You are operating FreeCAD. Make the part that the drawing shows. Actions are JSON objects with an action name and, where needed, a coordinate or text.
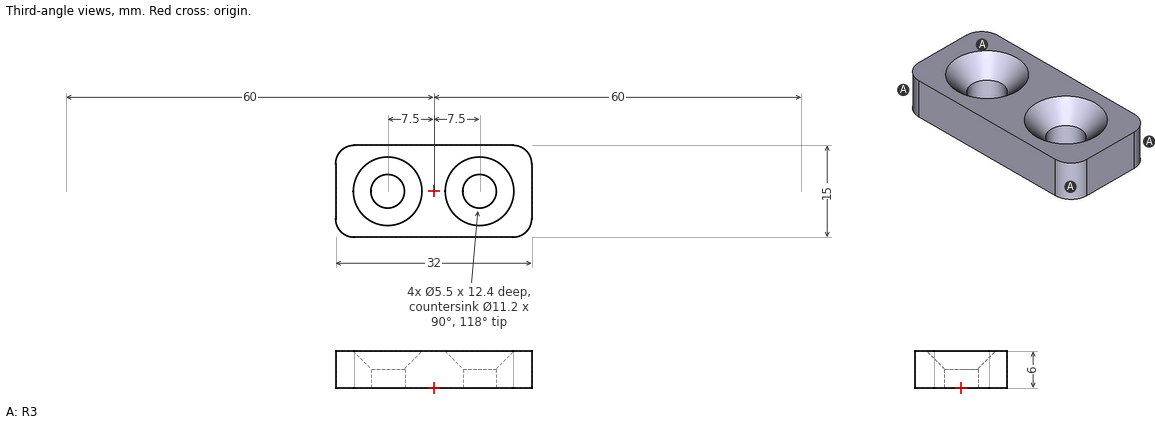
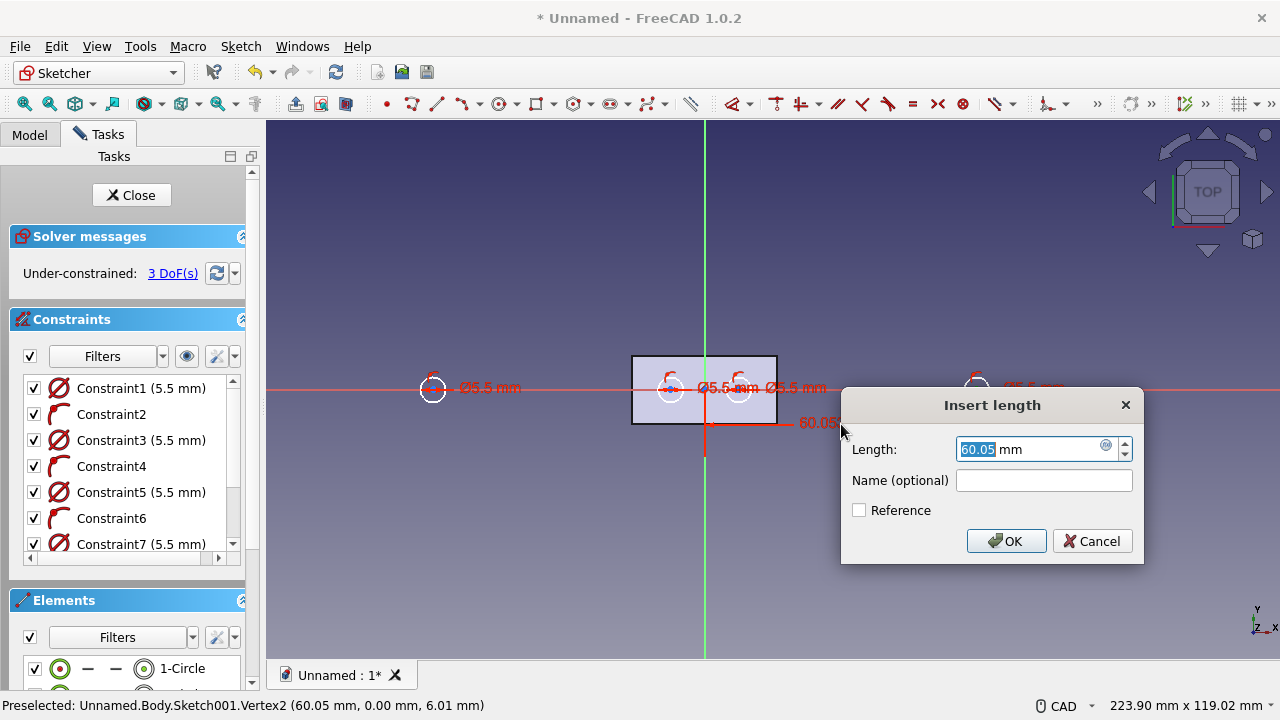
{"action": "type", "text": "60"}
{"action": "key", "text": "Return"}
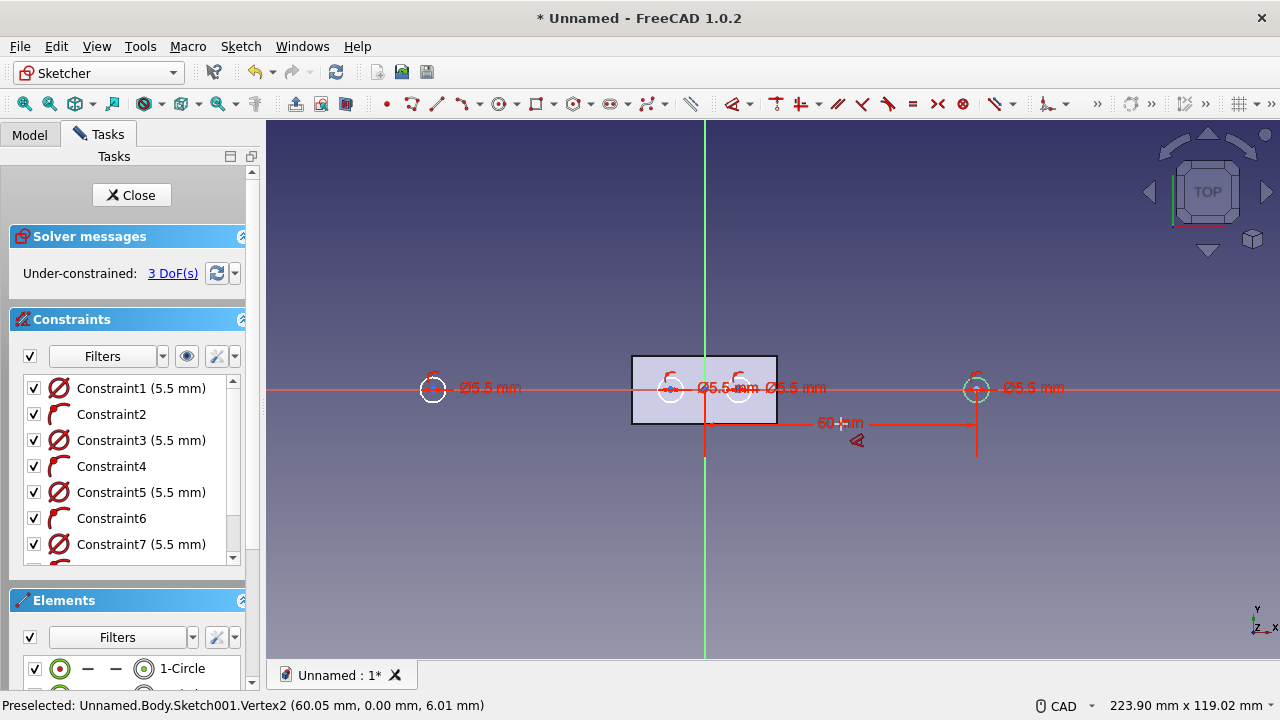
{"action": "left_click", "coordinate": [433, 390]}
{"action": "left_click", "coordinate": [569, 424]}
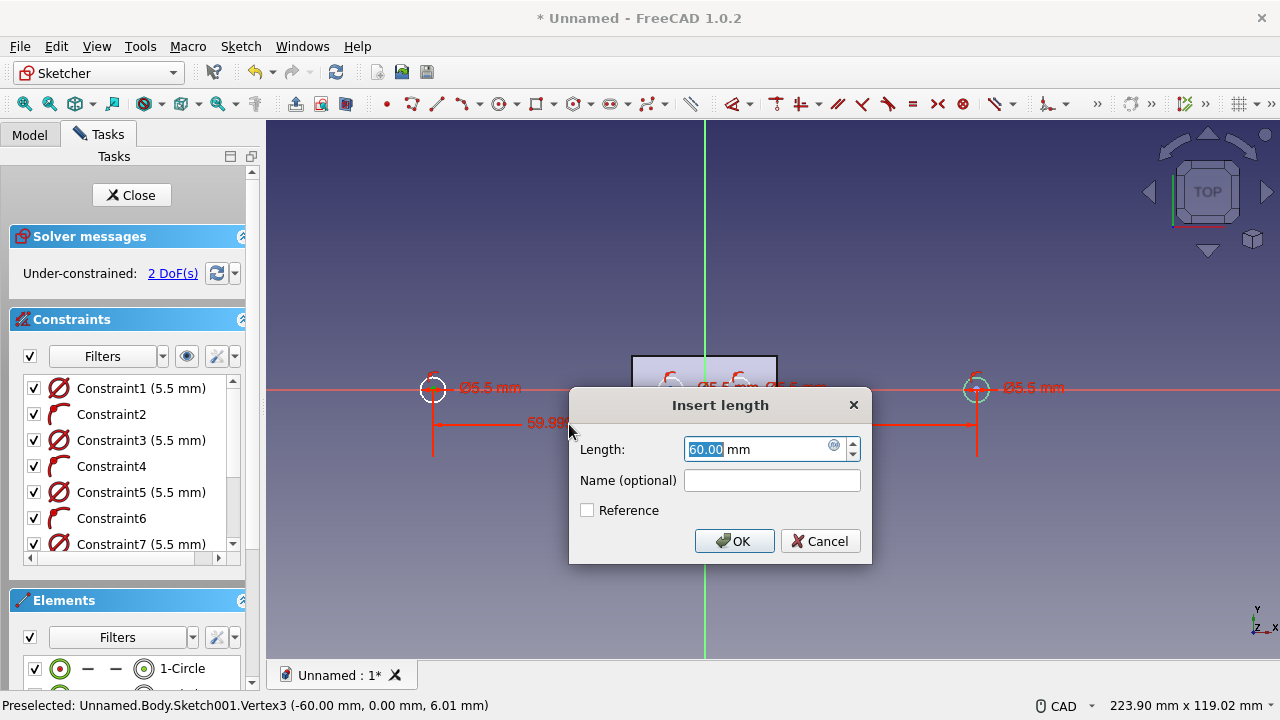
{"action": "type", "text": "60"}
{"action": "key", "text": "Return"}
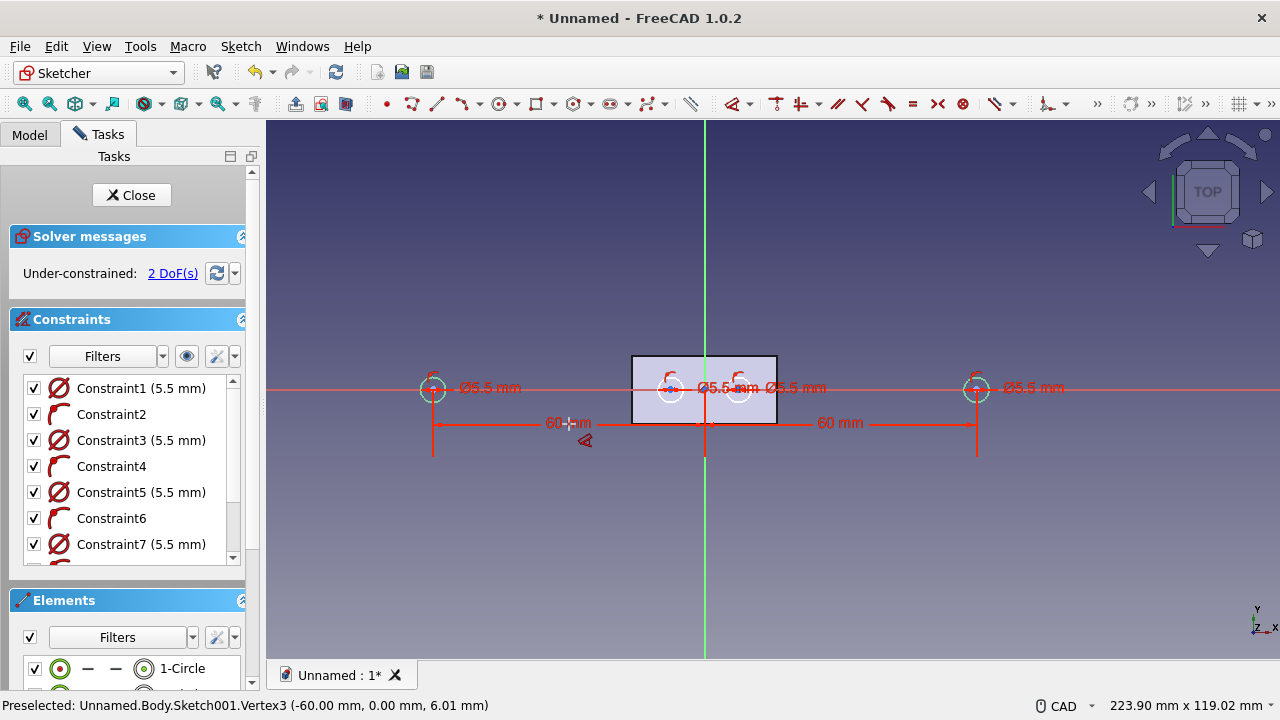
{"action": "left_click", "coordinate": [739, 390]}
{"action": "left_click", "coordinate": [722, 424]}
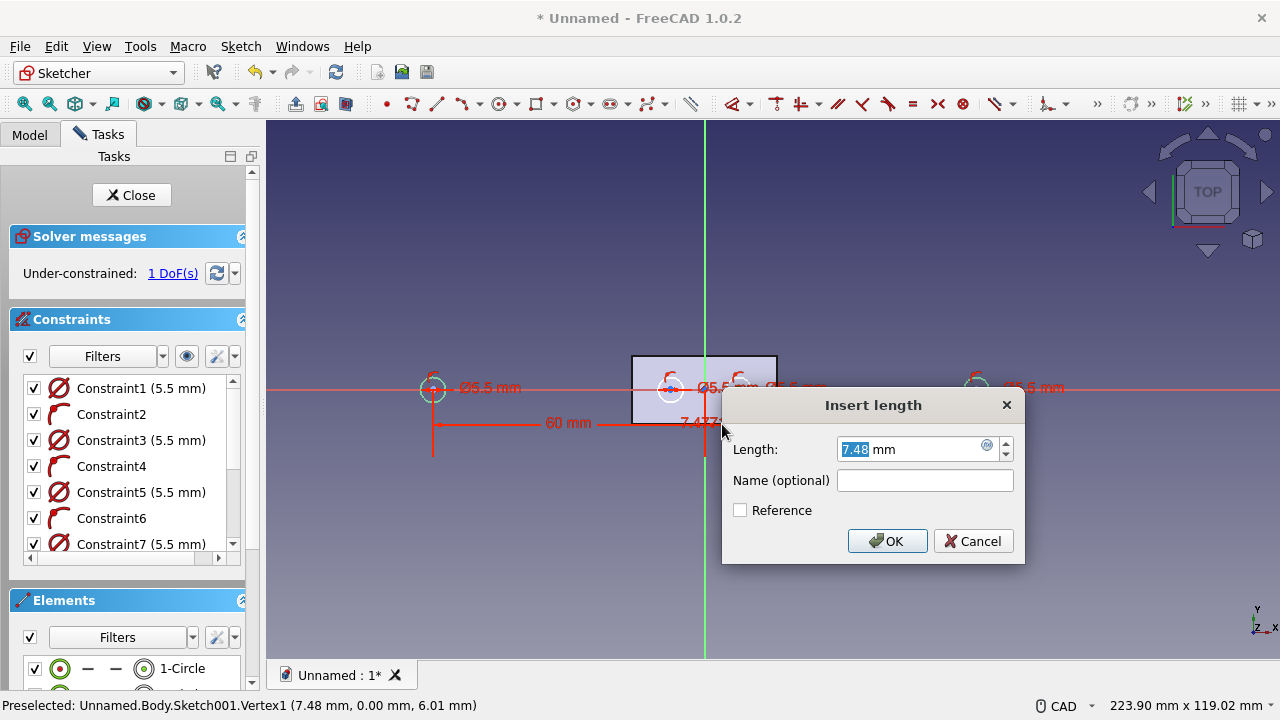
{"action": "type", "text": "7.5"}
{"action": "key", "text": "Return"}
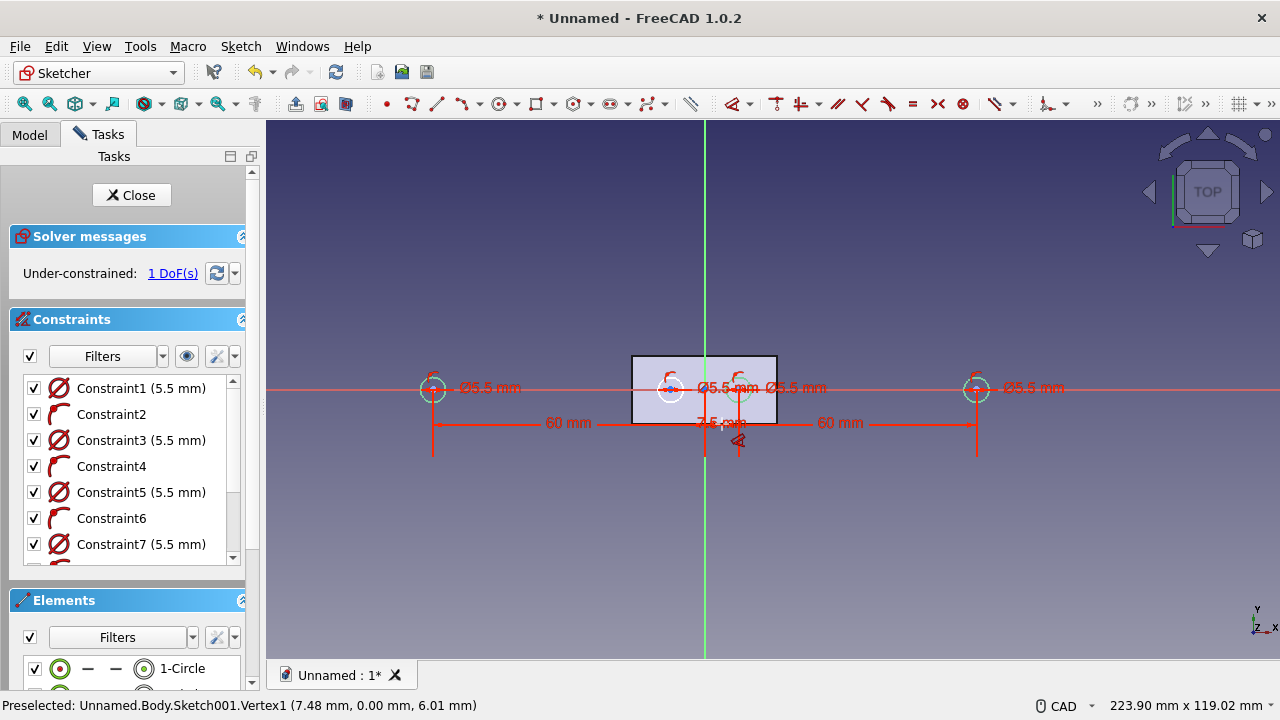
{"action": "left_click", "coordinate": [671, 390]}
{"action": "left_click", "coordinate": [688, 356]}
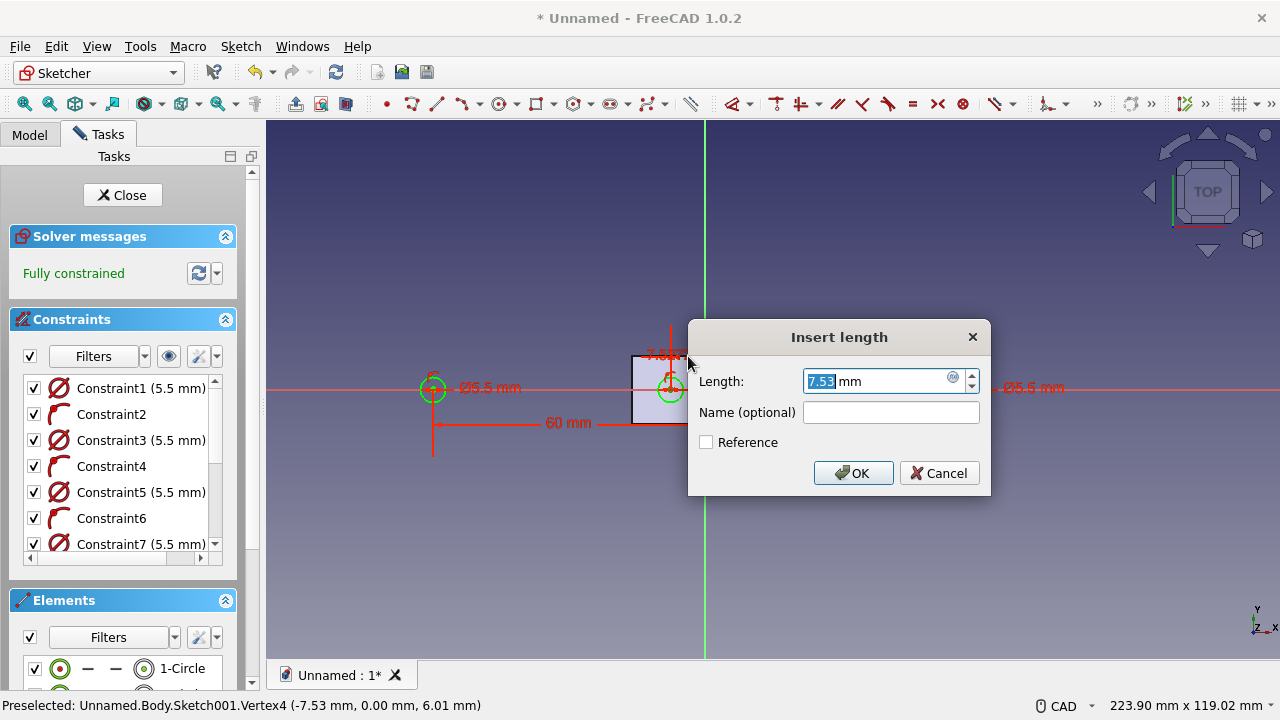
{"action": "type", "text": "7.5"}
{"action": "key", "text": "Return"}
{"action": "key", "text": "Escape"}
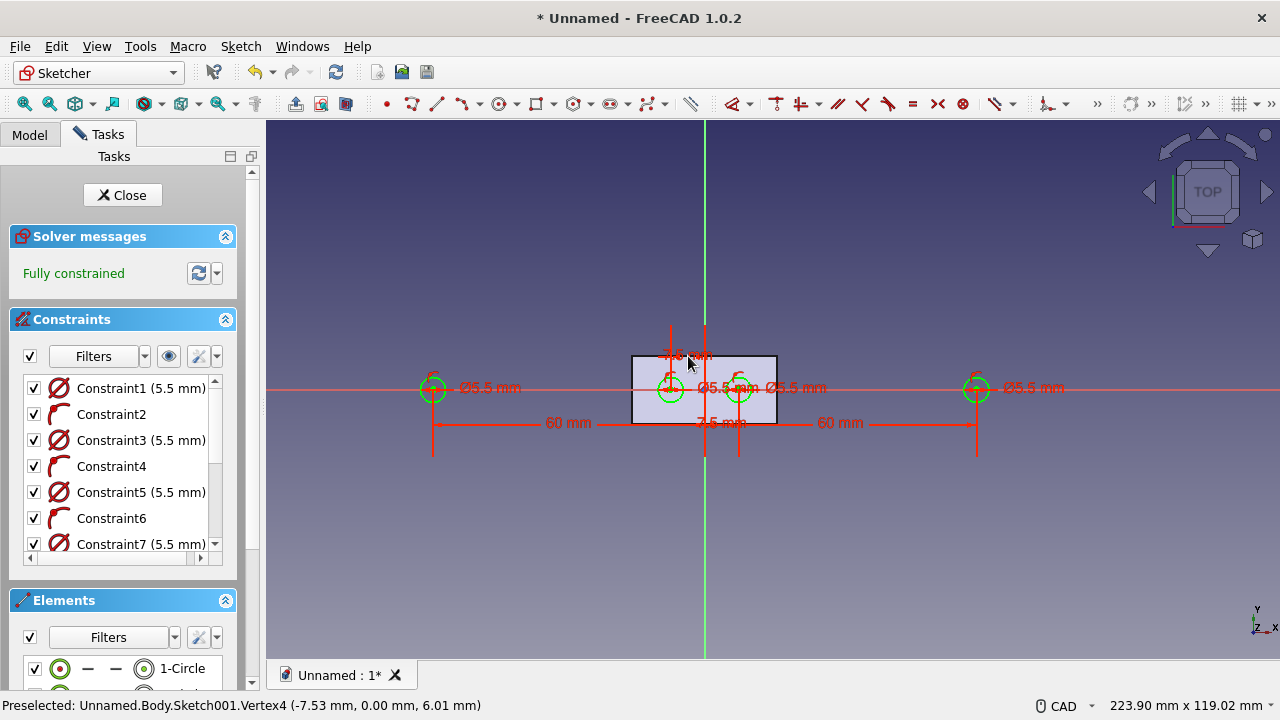
{"action": "left_click", "coordinate": [123, 195]}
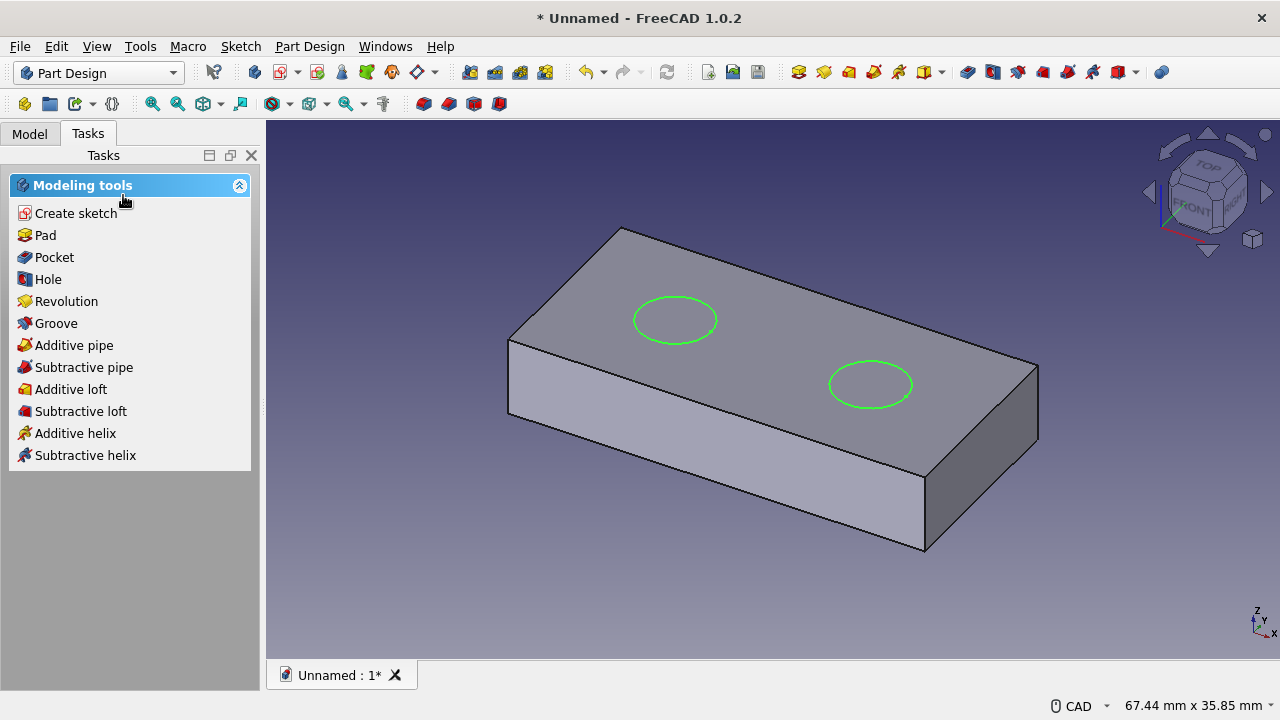
{"action": "left_click", "coordinate": [993, 72]}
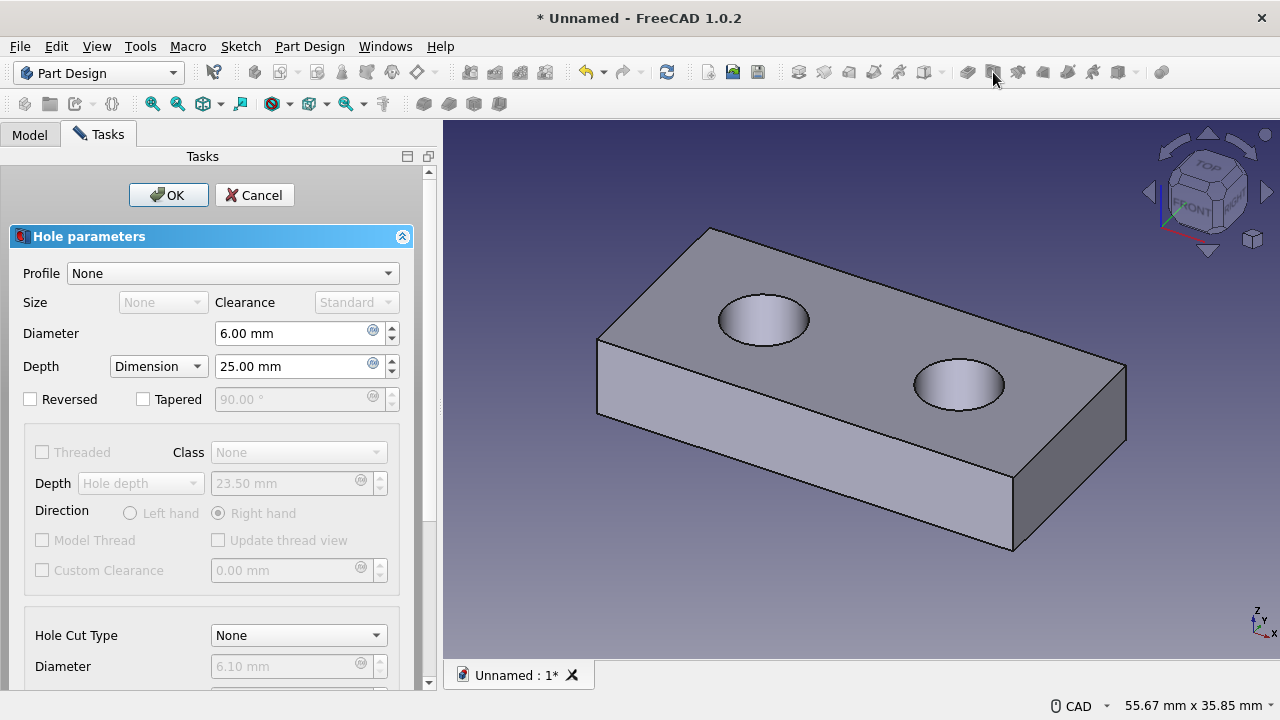
{"action": "triple_click", "coordinate": [300, 334]}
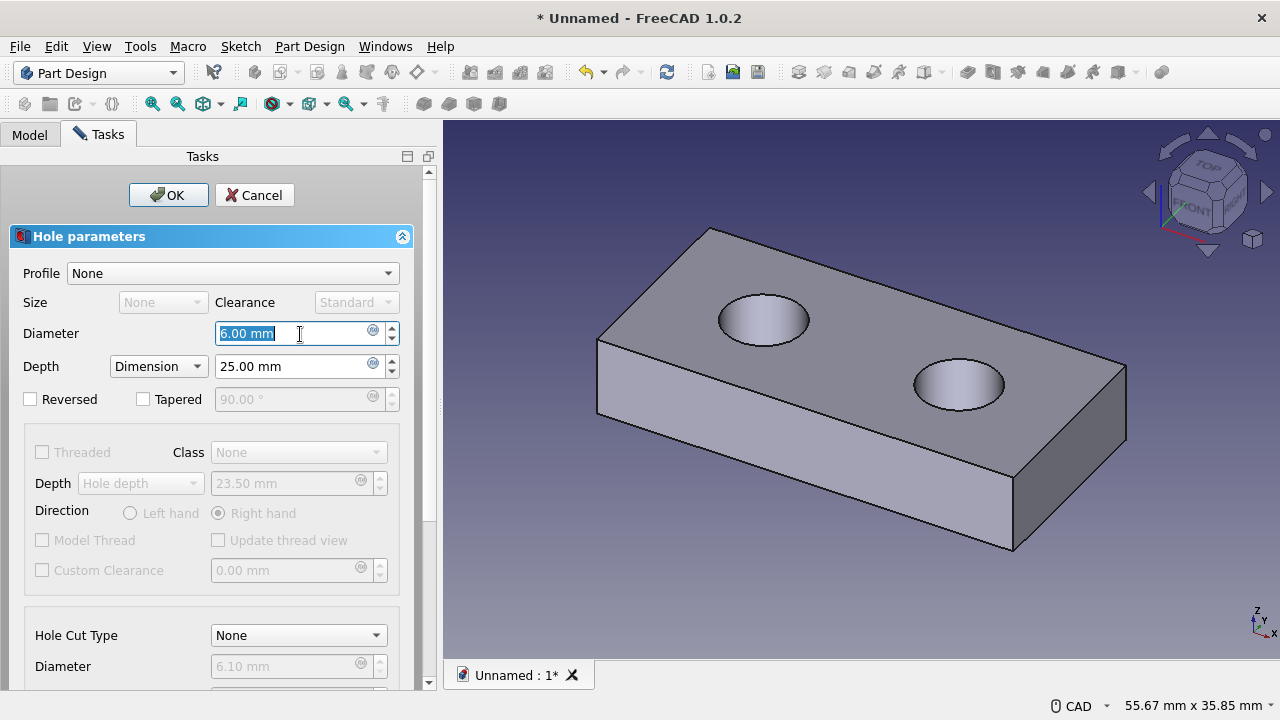
{"action": "type", "text": "5.5"}
{"action": "key", "text": "Tab"}